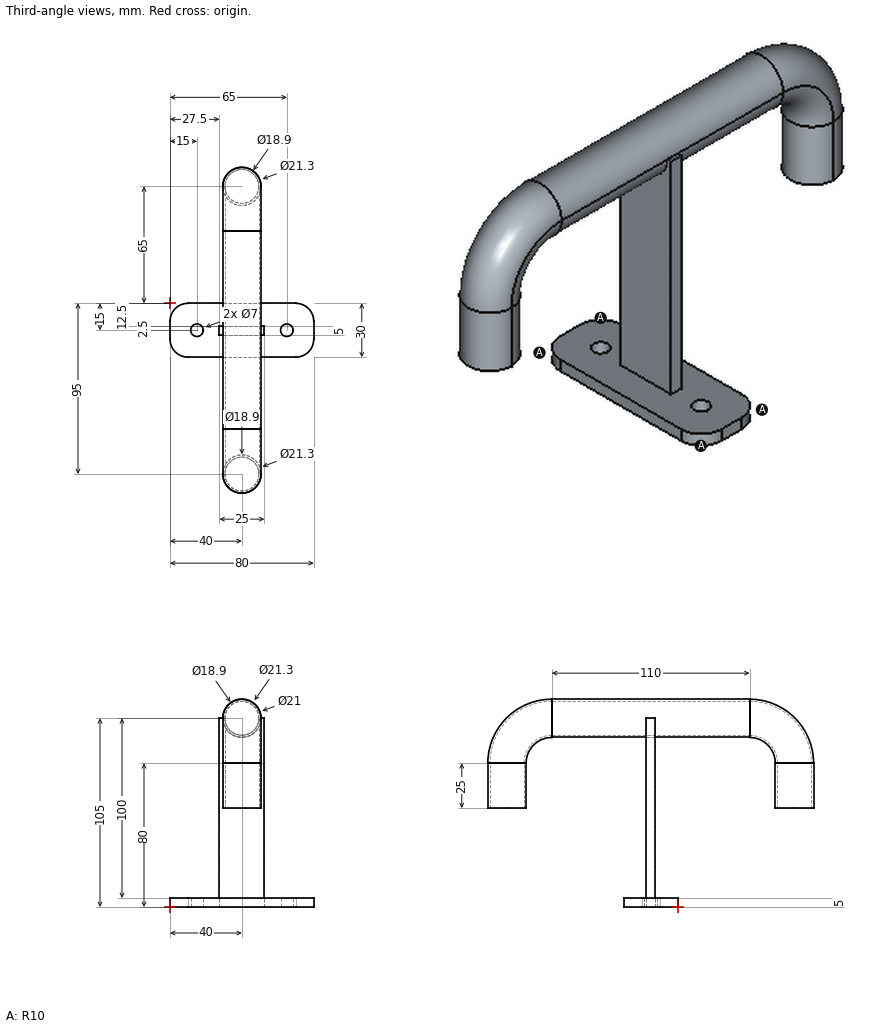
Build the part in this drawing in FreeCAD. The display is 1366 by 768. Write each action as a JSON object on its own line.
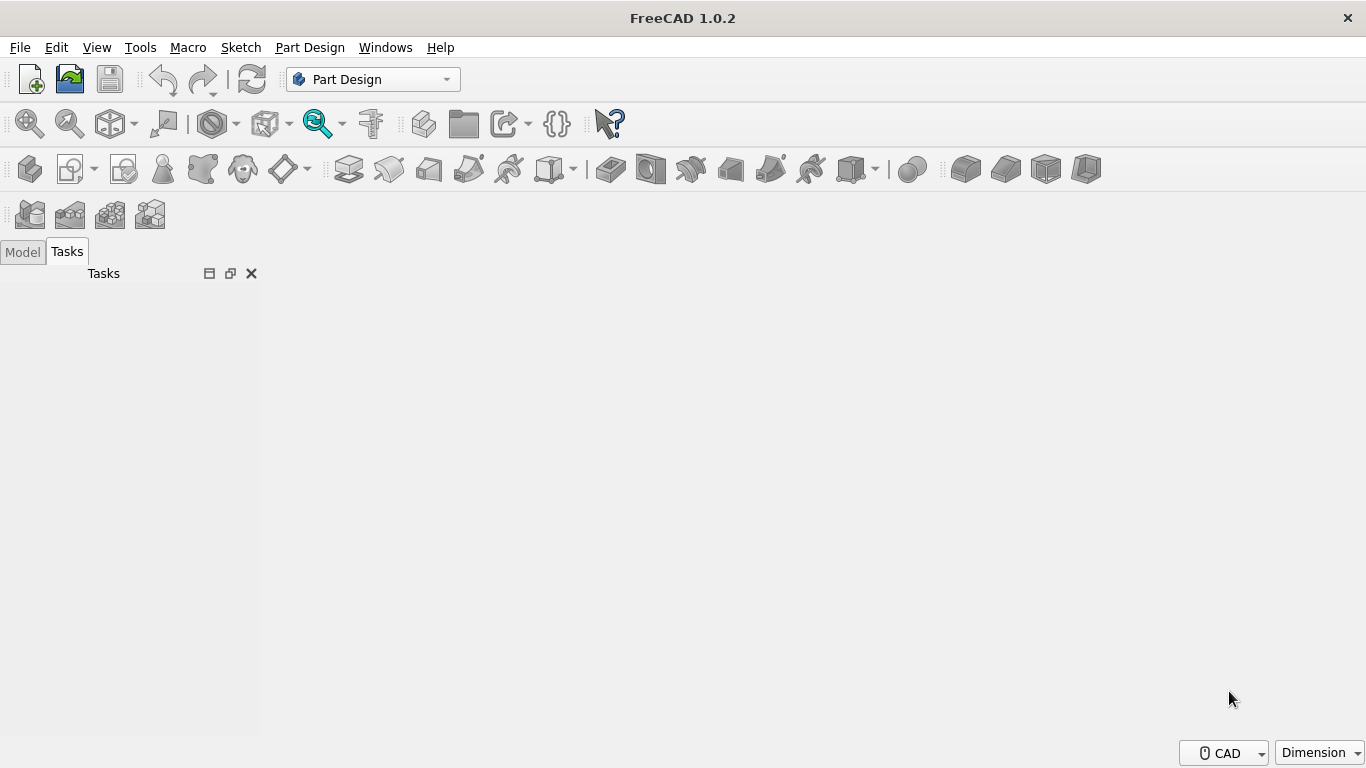
{"action": "left_click", "coordinate": [30, 80]}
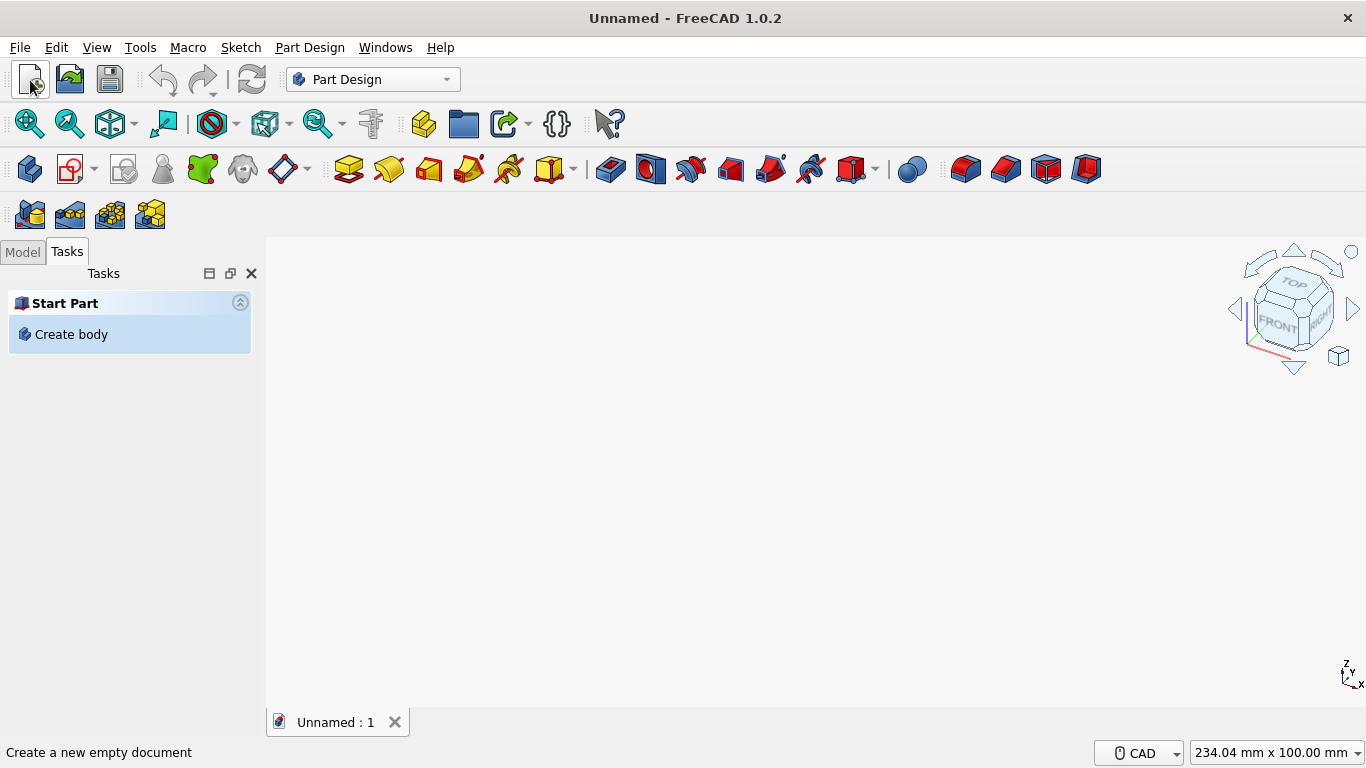
{"action": "left_click", "coordinate": [70, 170]}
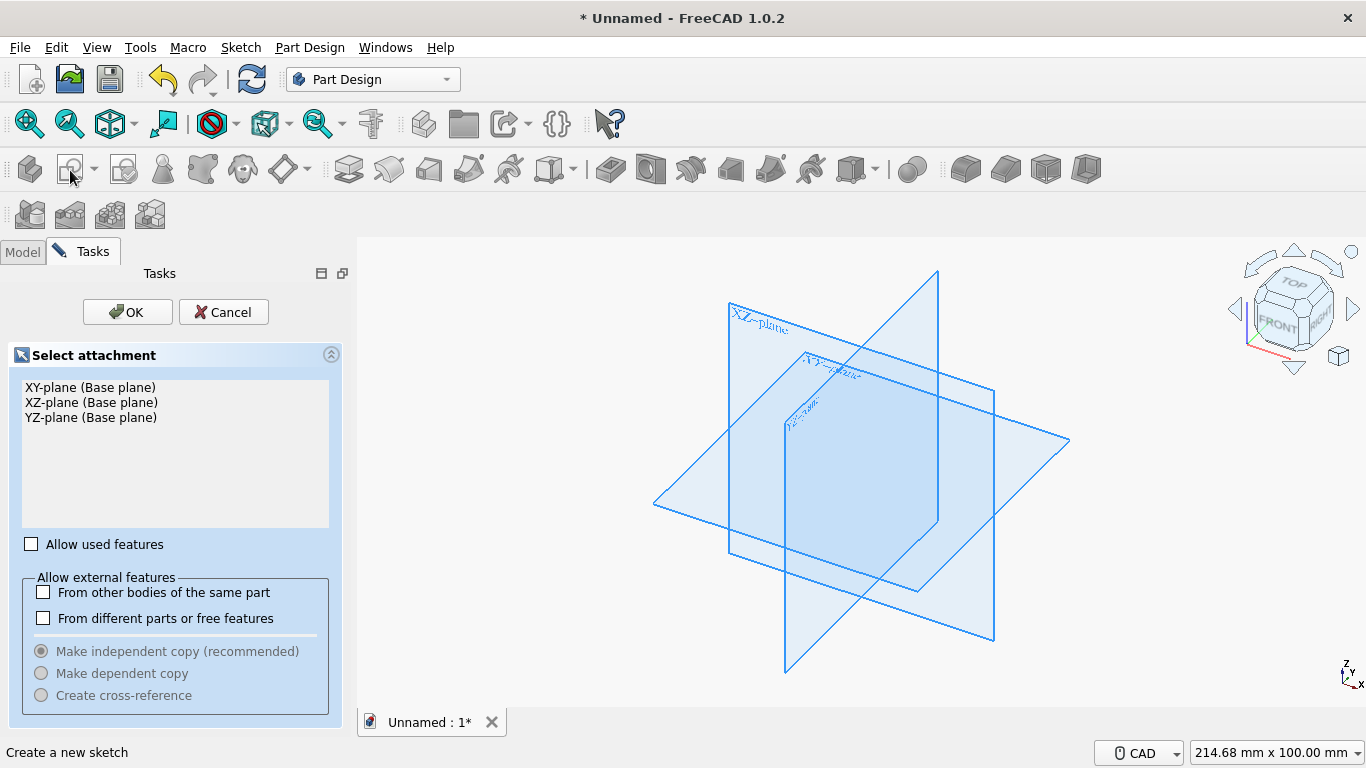
{"action": "left_click", "coordinate": [82, 388]}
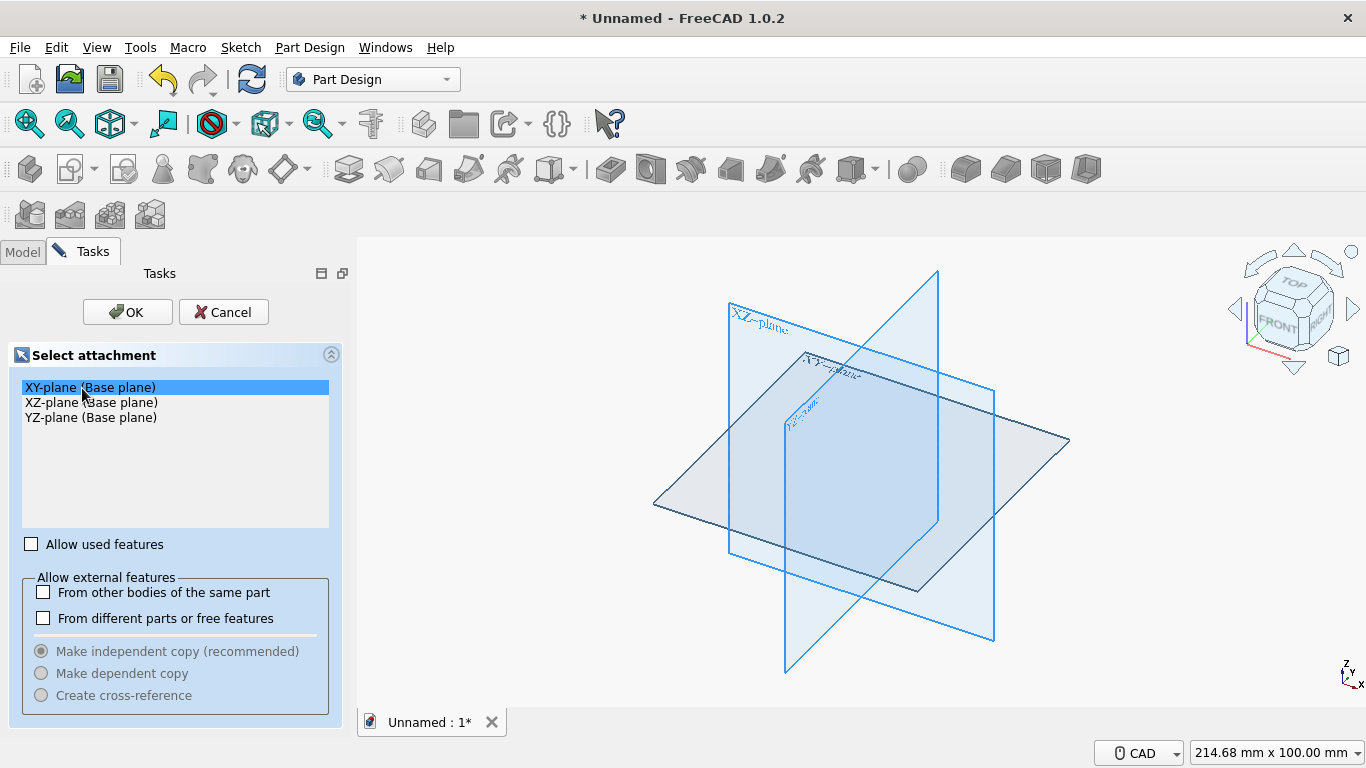
{"action": "left_click", "coordinate": [128, 312]}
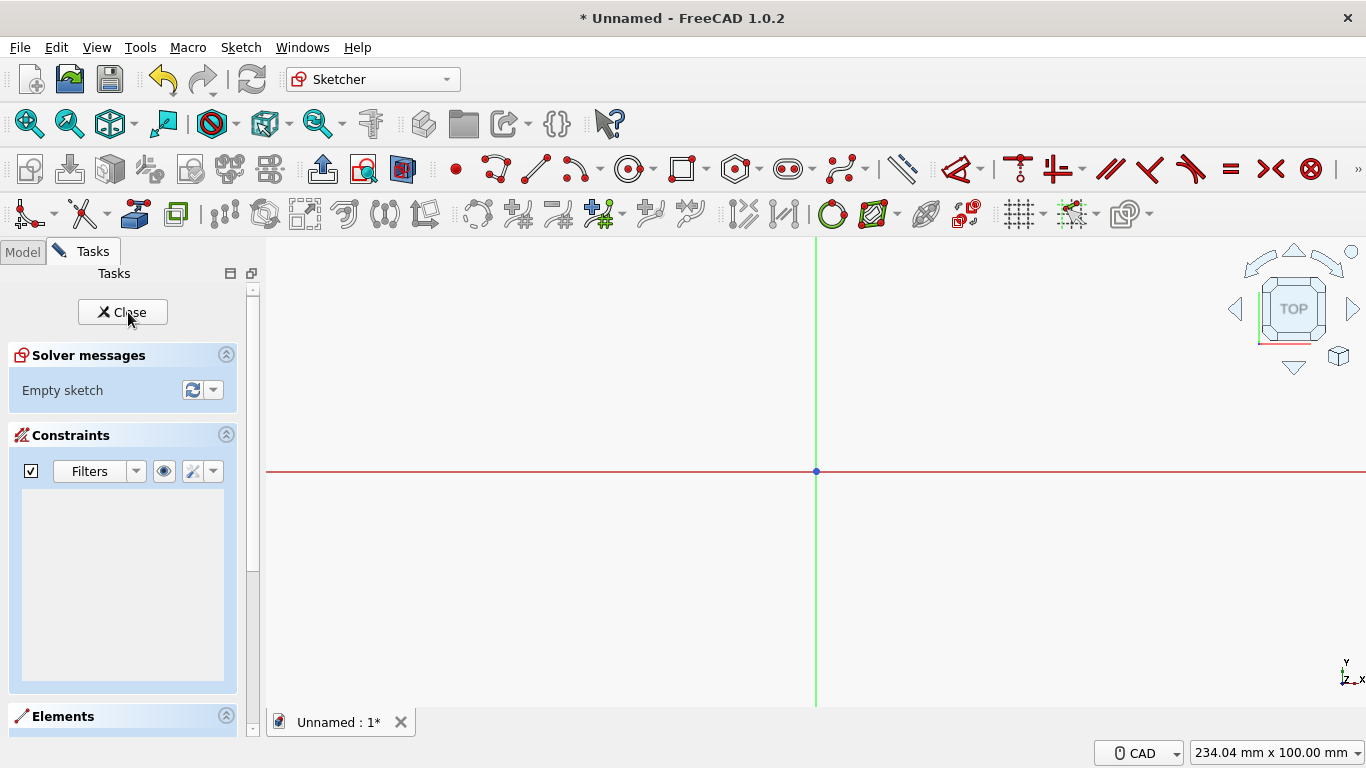
{"action": "scroll", "coordinate": [748, 472], "scroll_direction": "down", "scroll_amount": 5}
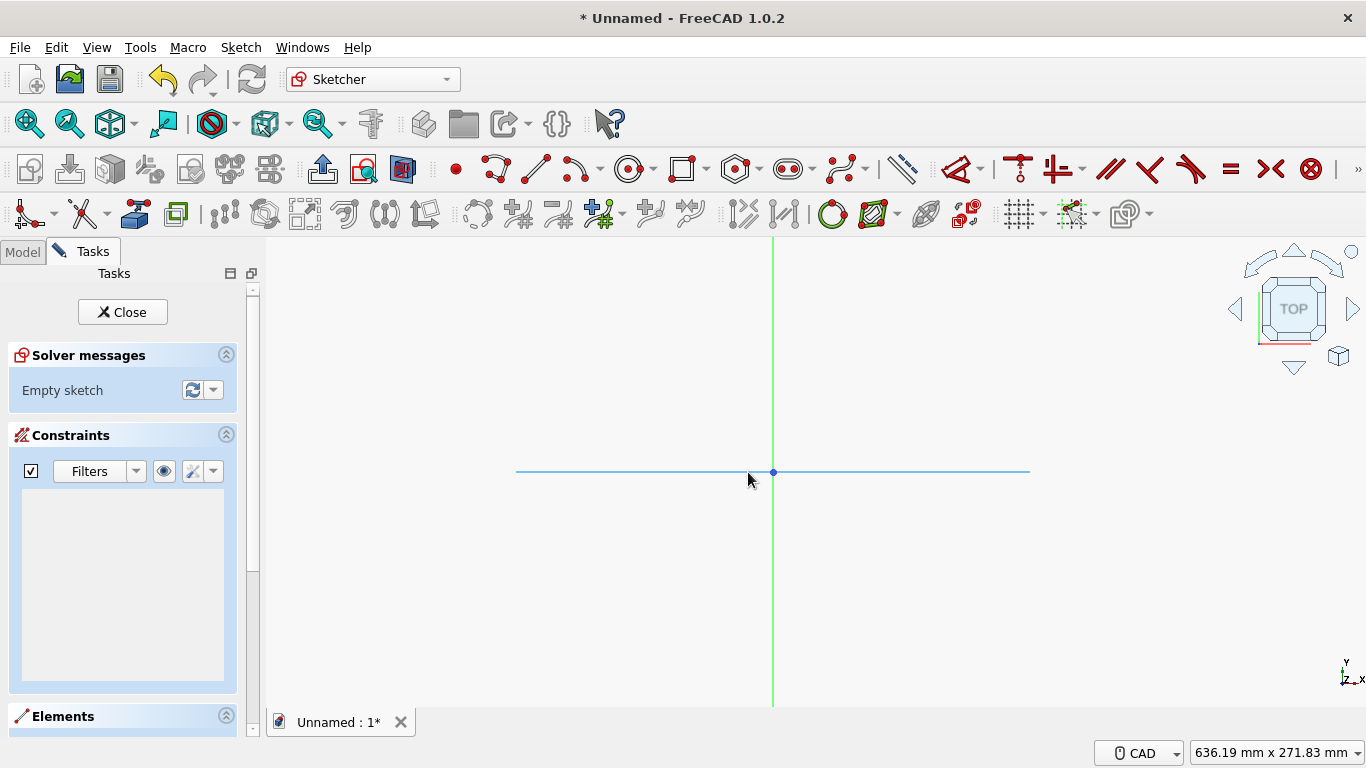
{"action": "scroll", "coordinate": [866, 505], "scroll_direction": "up", "scroll_amount": 8}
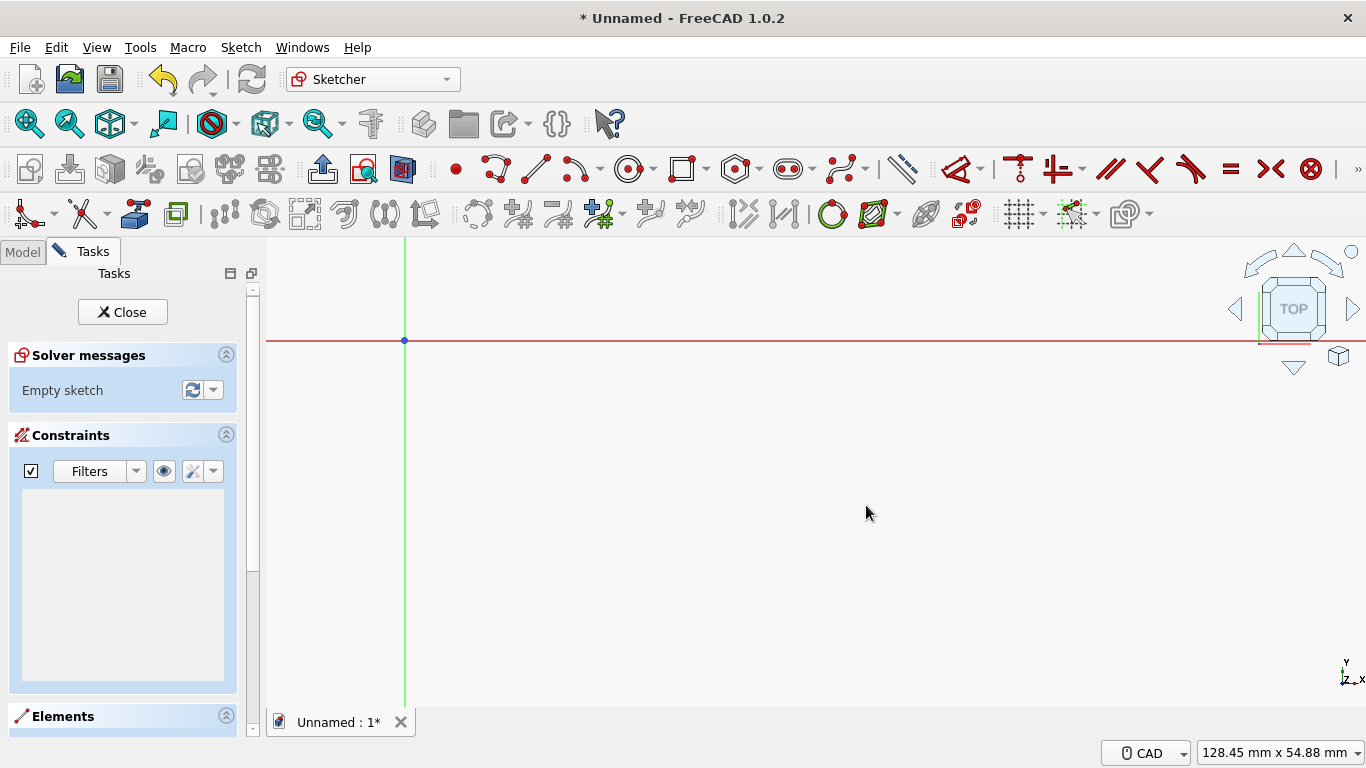
{"action": "left_click", "coordinate": [682, 170]}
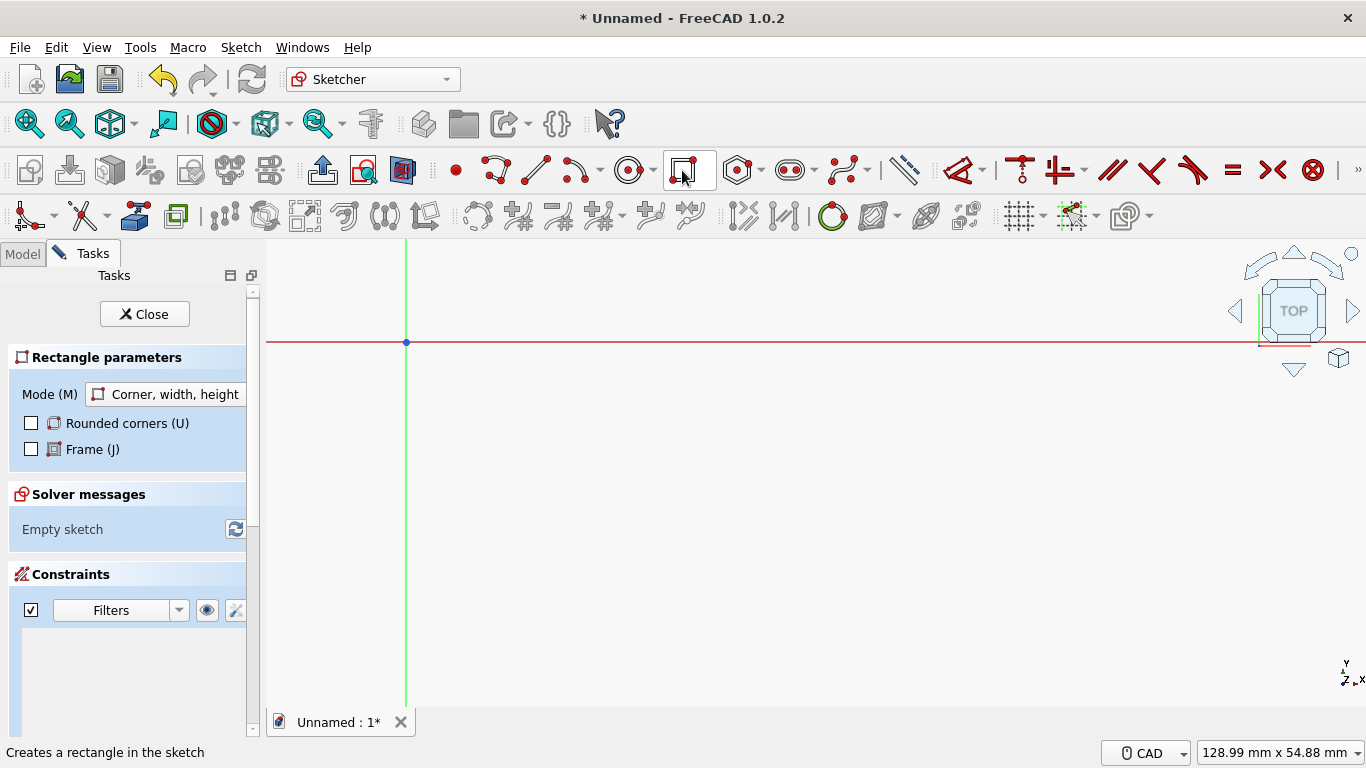
{"action": "left_click", "coordinate": [406, 342]}
{"action": "mouse_move", "coordinate": [1089, 598]}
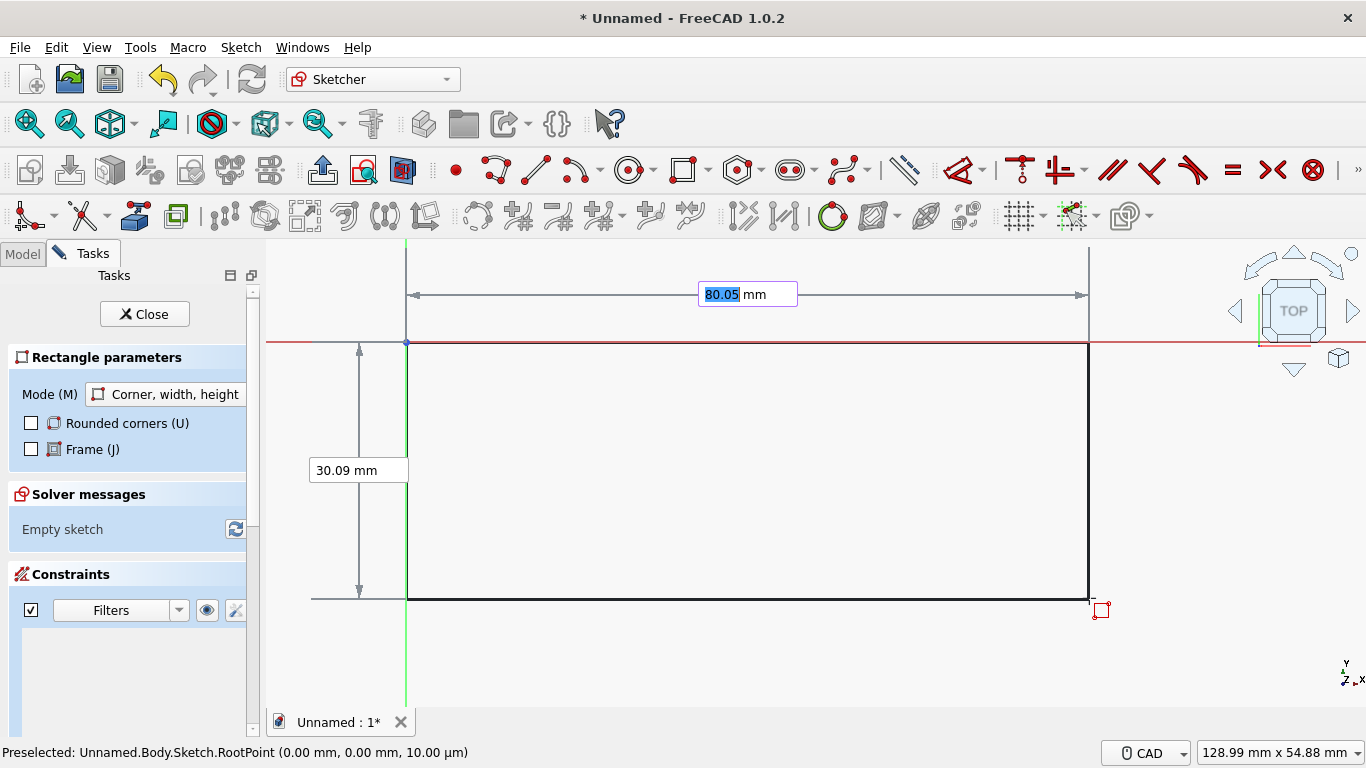
{"action": "type", "text": "80"}
{"action": "key", "text": "Tab"}
{"action": "type", "text": "30"}
{"action": "key", "text": "Return"}